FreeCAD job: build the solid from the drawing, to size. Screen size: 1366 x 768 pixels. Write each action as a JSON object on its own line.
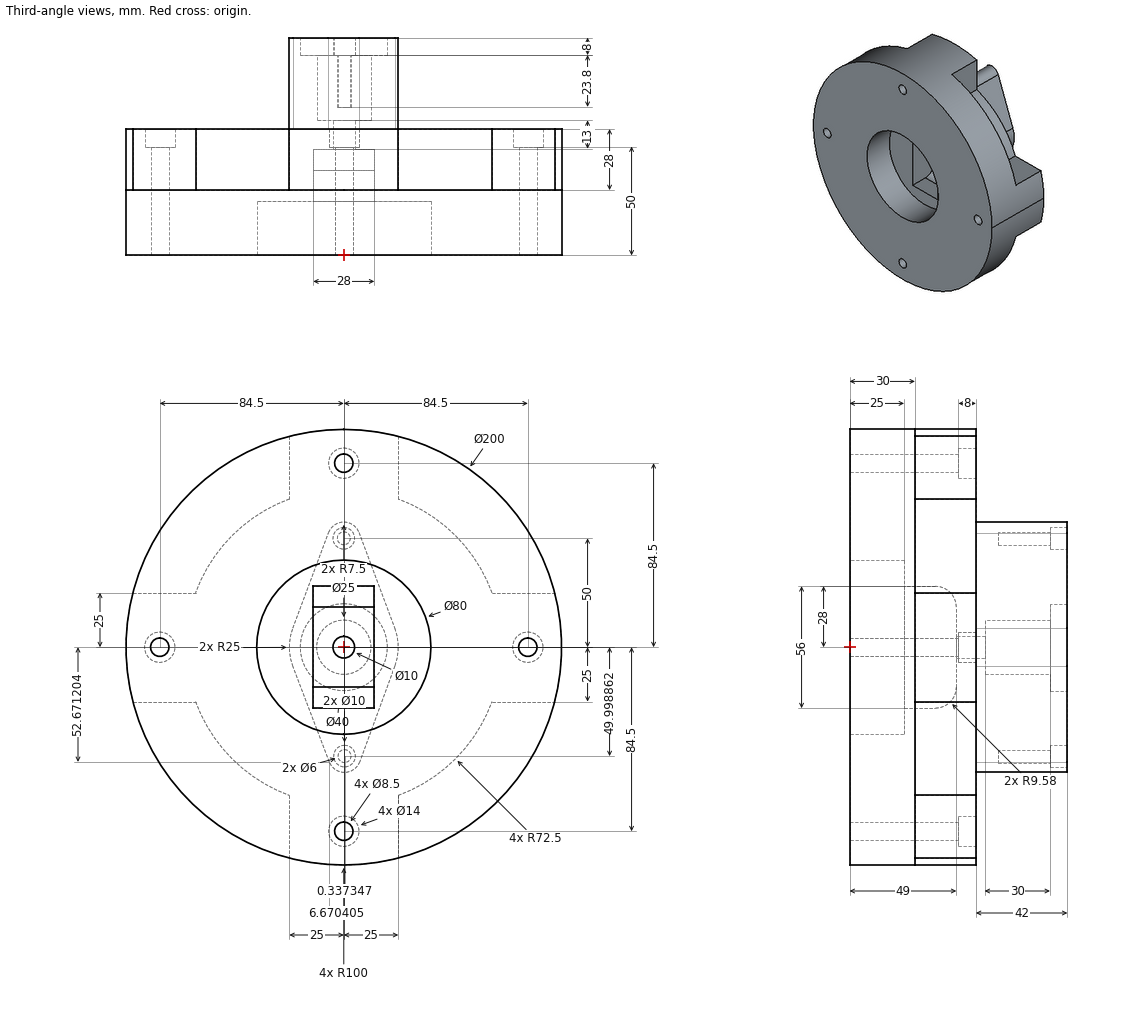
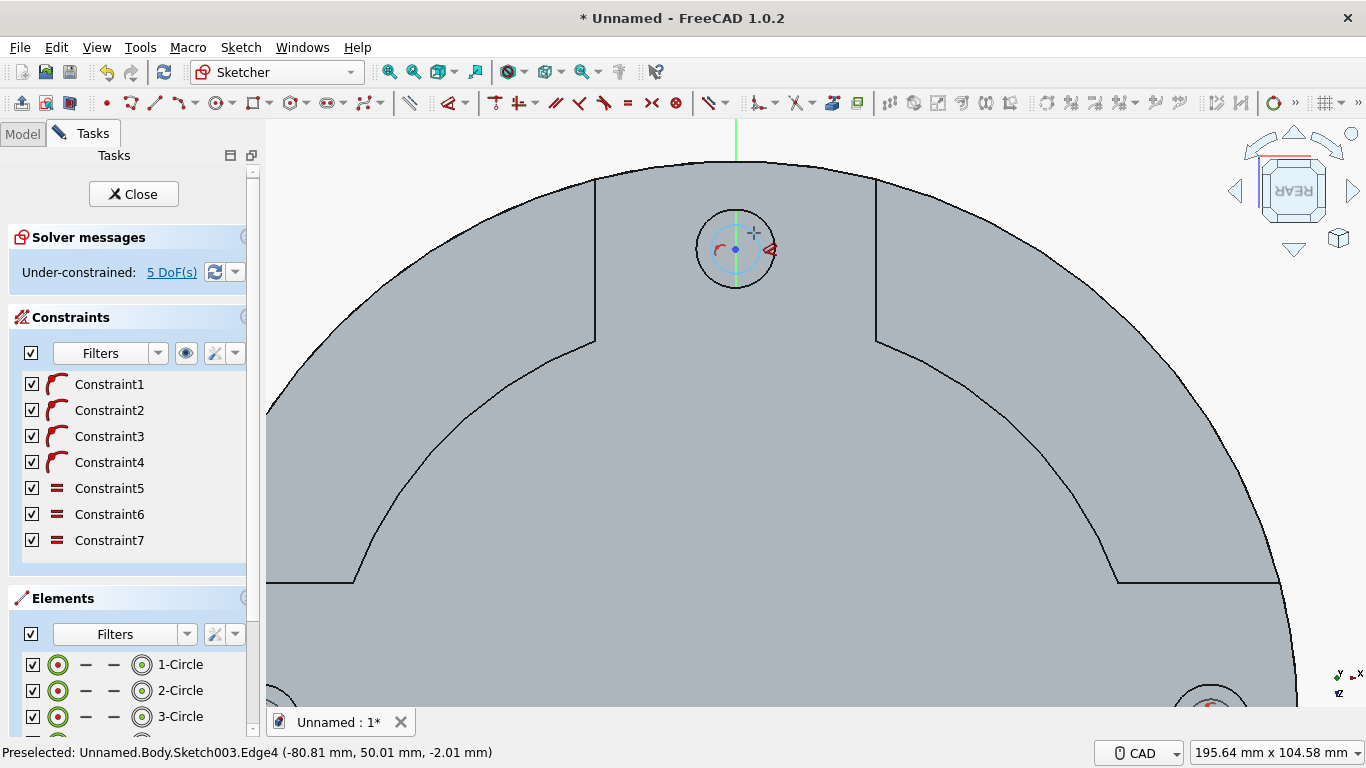
{"action": "left_click", "coordinate": [753, 232]}
{"action": "left_click", "coordinate": [776, 209]}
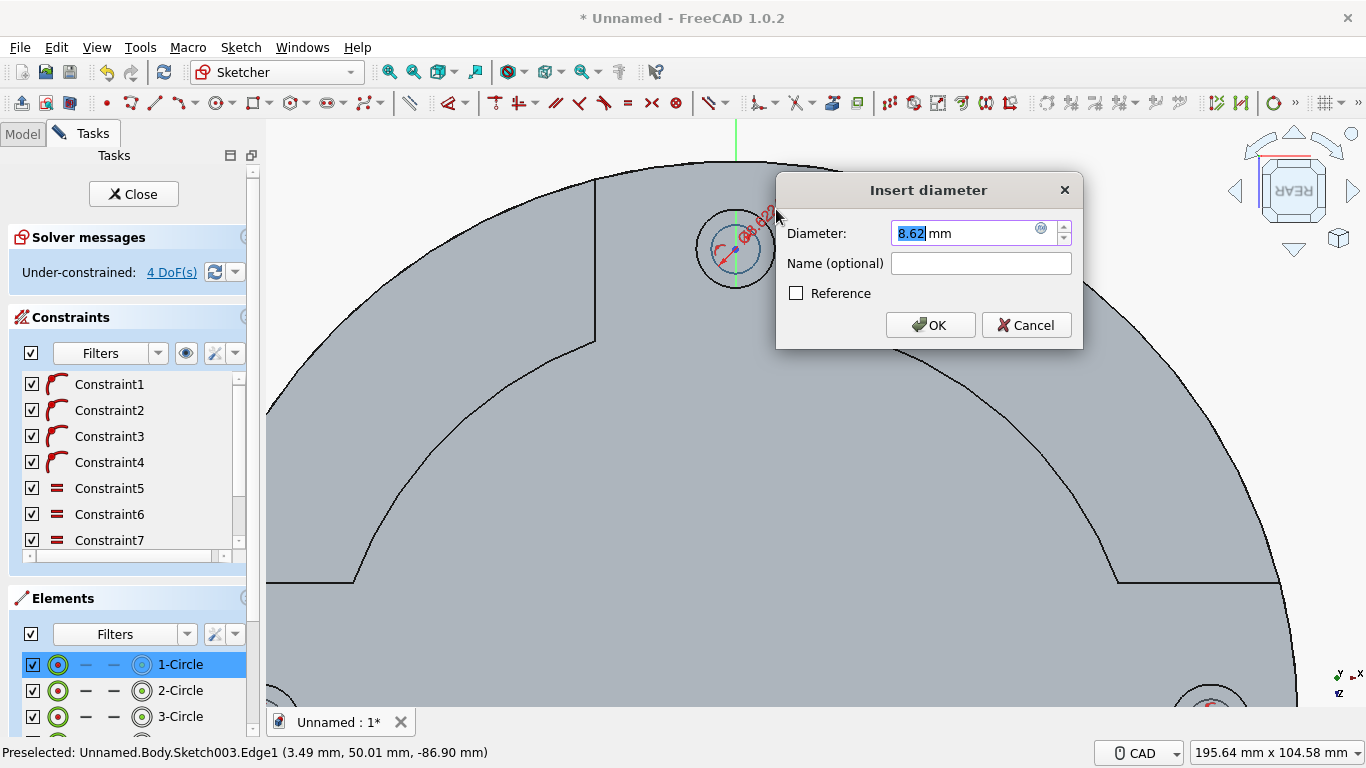
{"action": "type", "text": "8.5"}
{"action": "key", "text": "Return"}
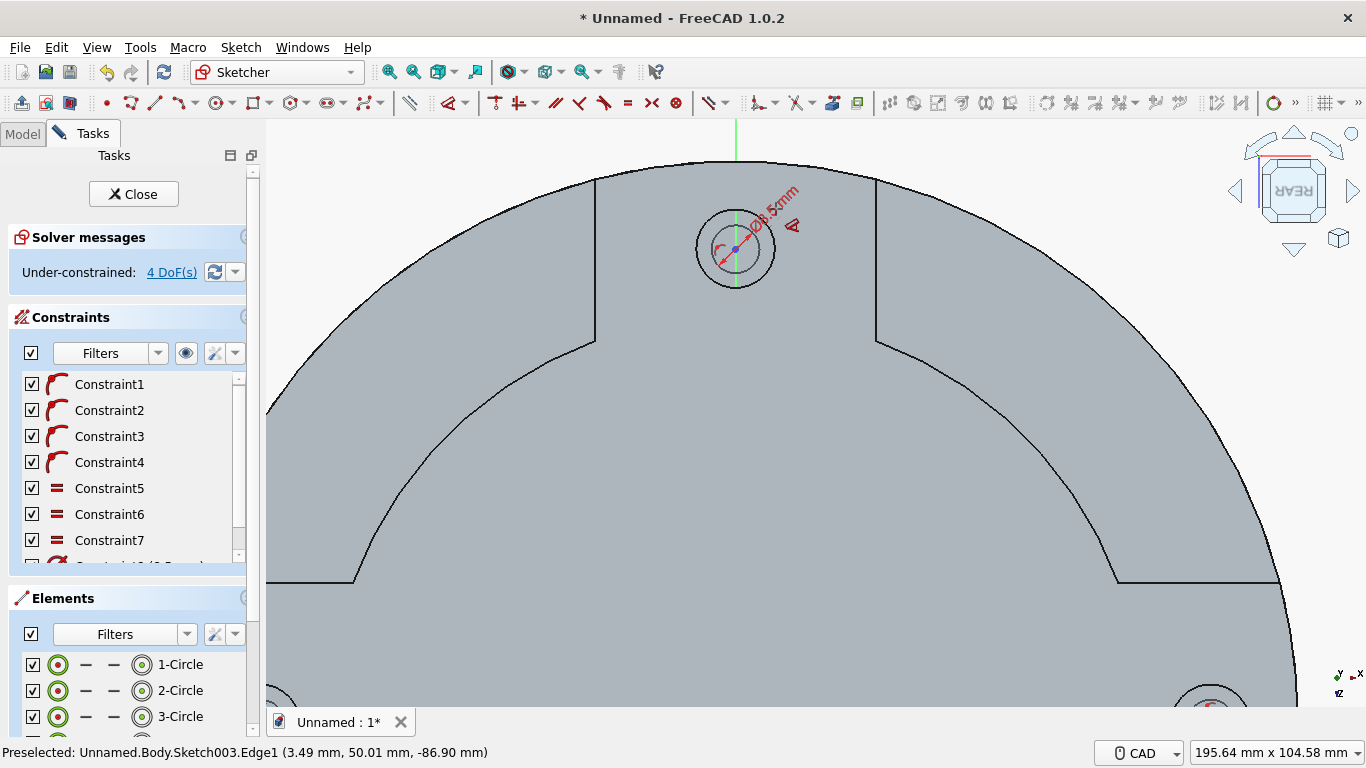
{"action": "left_click", "coordinate": [736, 249]}
{"action": "left_click", "coordinate": [770, 464]}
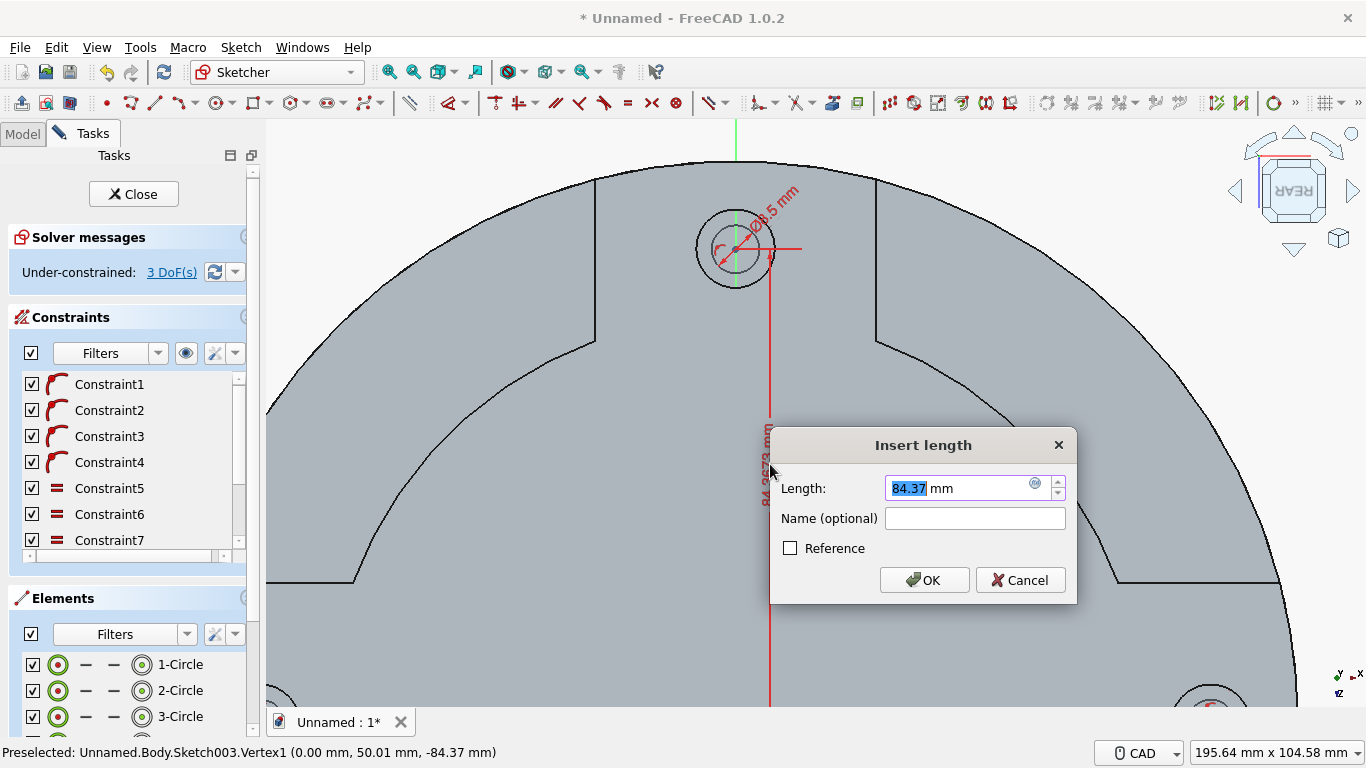
{"action": "type", "text": "84.5"}
{"action": "key", "text": "Return"}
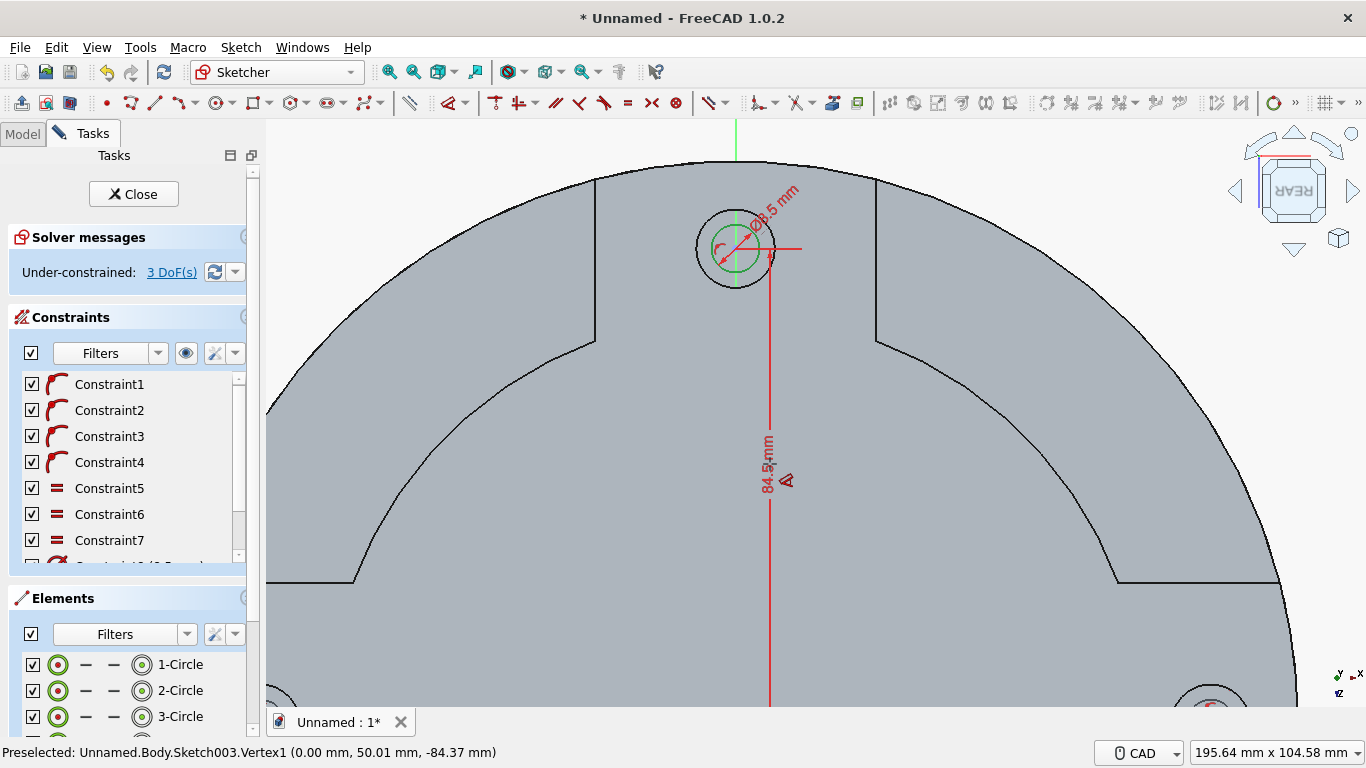
{"action": "scroll", "coordinate": [754, 232], "scroll_direction": "down", "scroll_amount": 5}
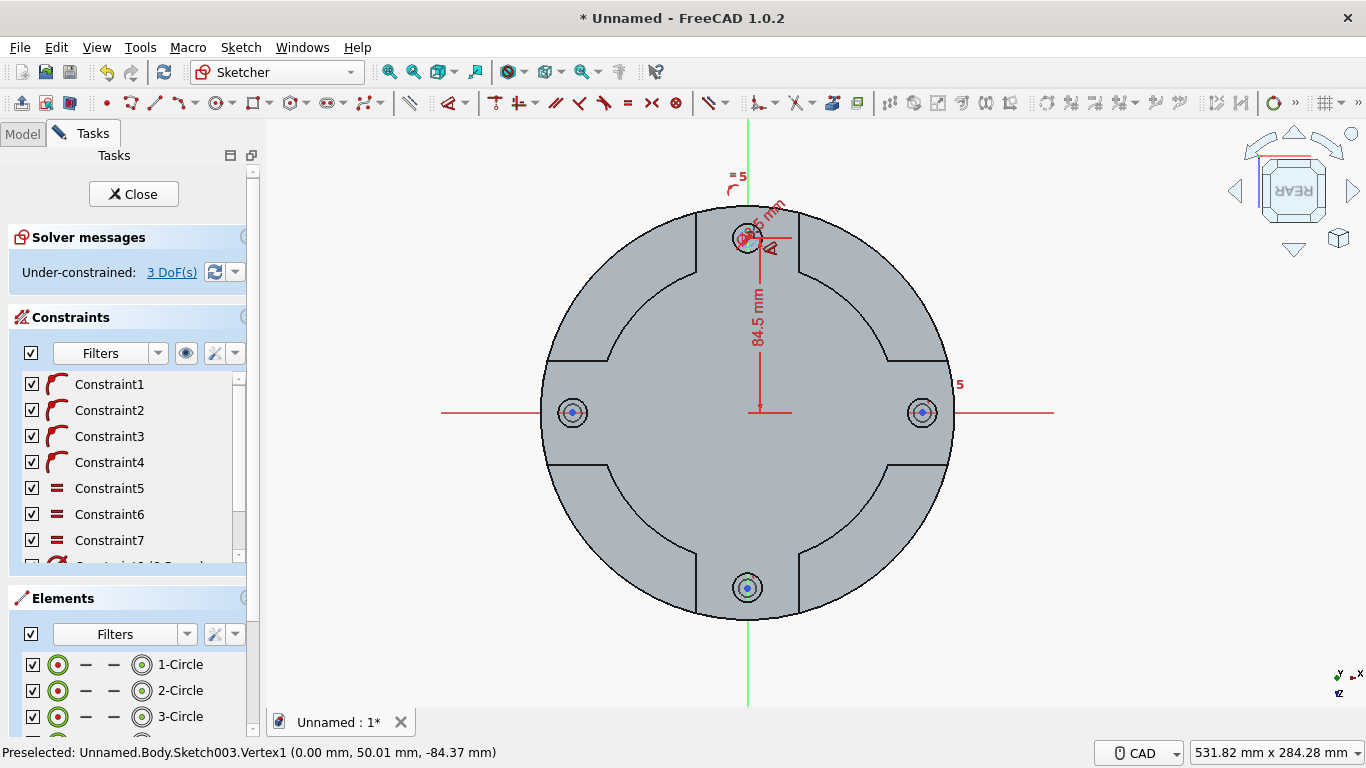
{"action": "left_click", "coordinate": [922, 413]}
{"action": "left_click", "coordinate": [835, 447]}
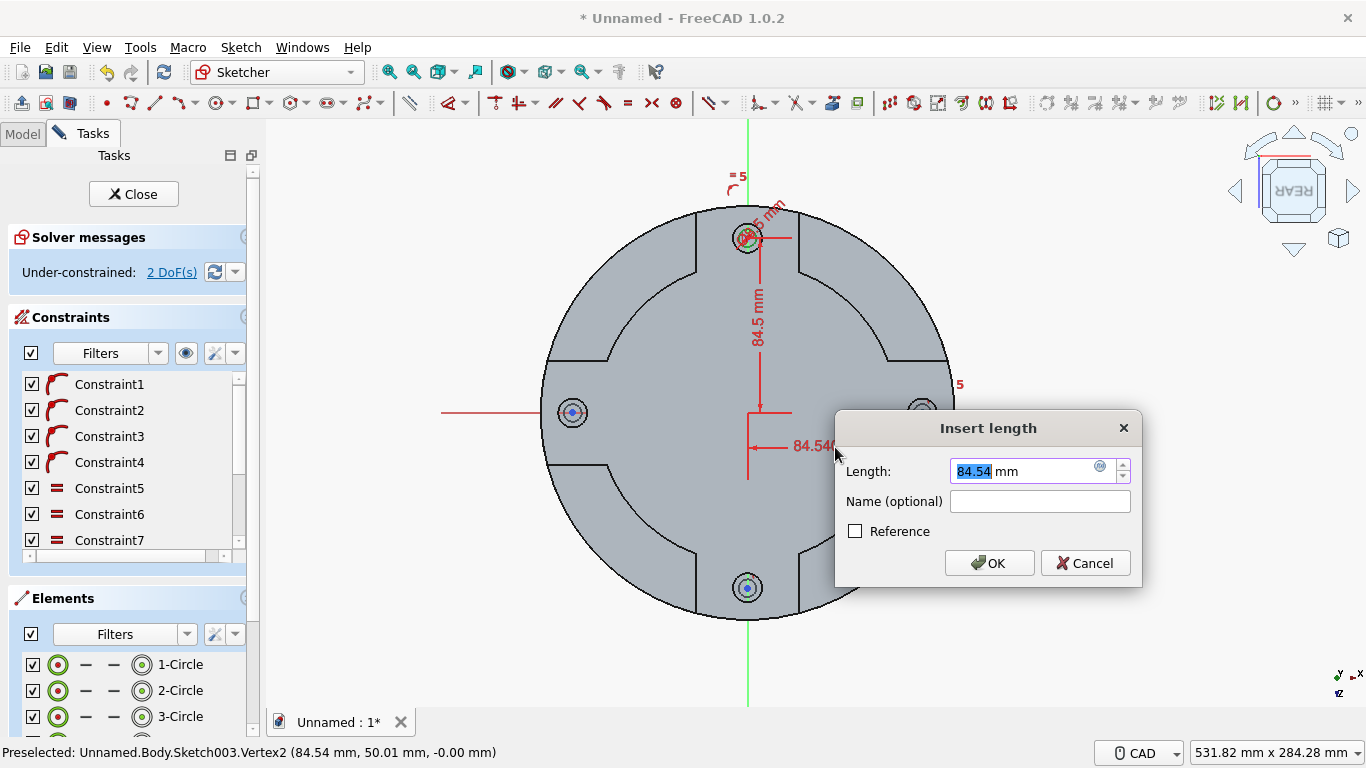
{"action": "type", "text": "84.5"}
{"action": "key", "text": "Return"}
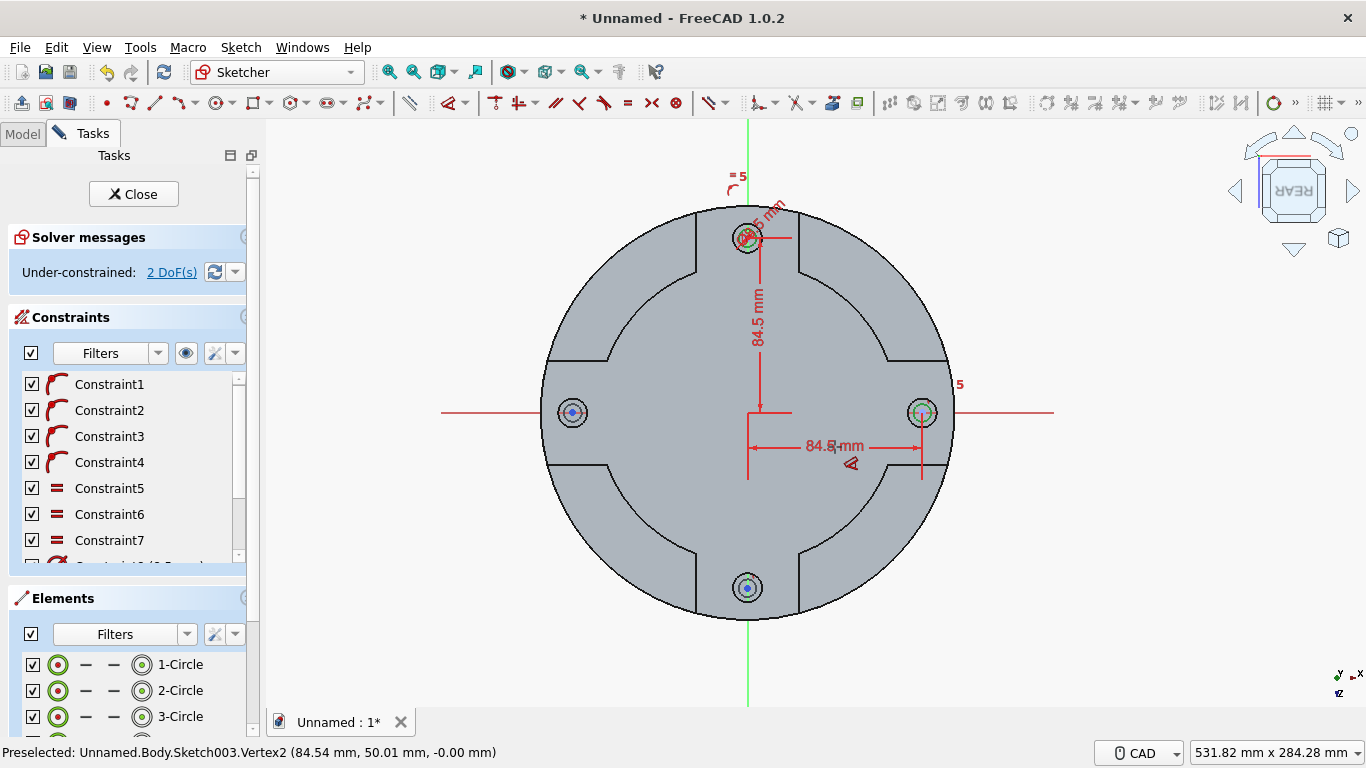
{"action": "left_click", "coordinate": [748, 588]}
{"action": "left_click", "coordinate": [782, 501]}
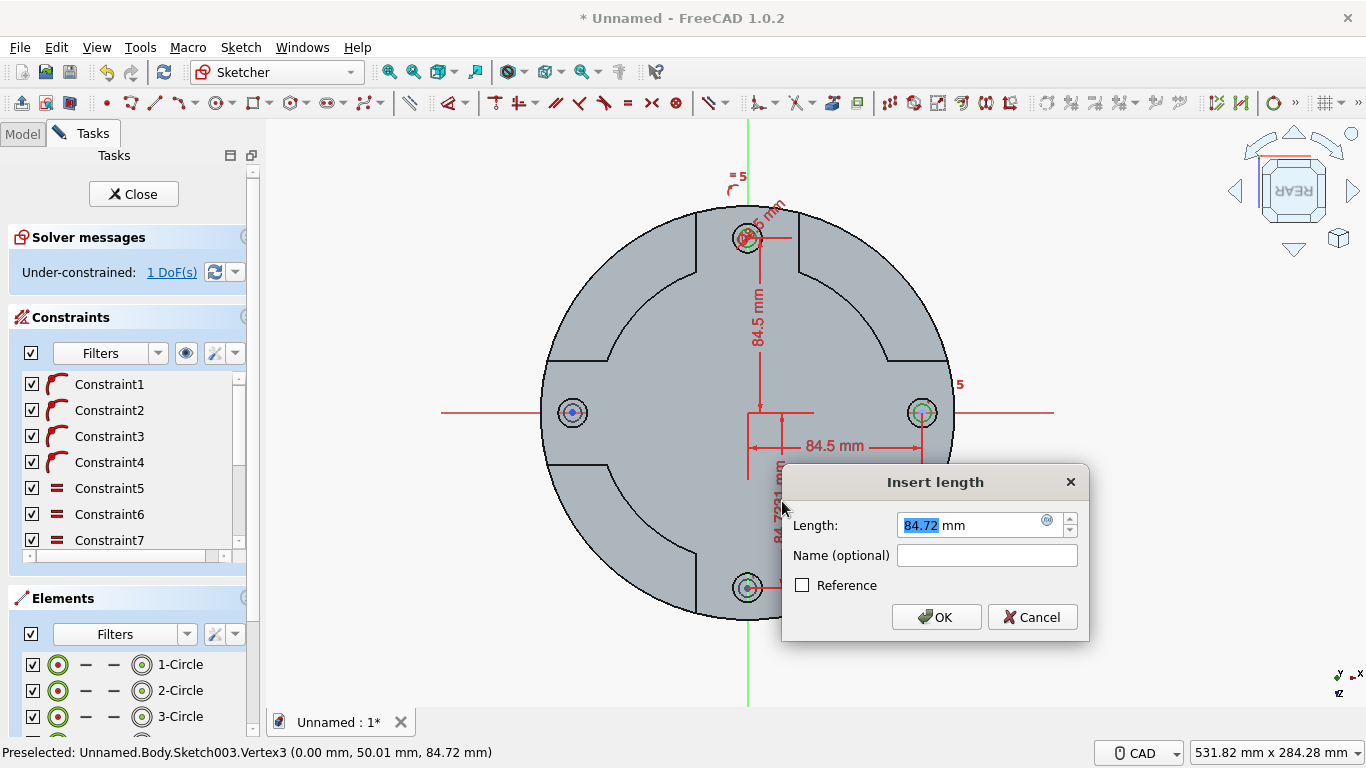
{"action": "type", "text": "84.5"}
{"action": "key", "text": "Return"}